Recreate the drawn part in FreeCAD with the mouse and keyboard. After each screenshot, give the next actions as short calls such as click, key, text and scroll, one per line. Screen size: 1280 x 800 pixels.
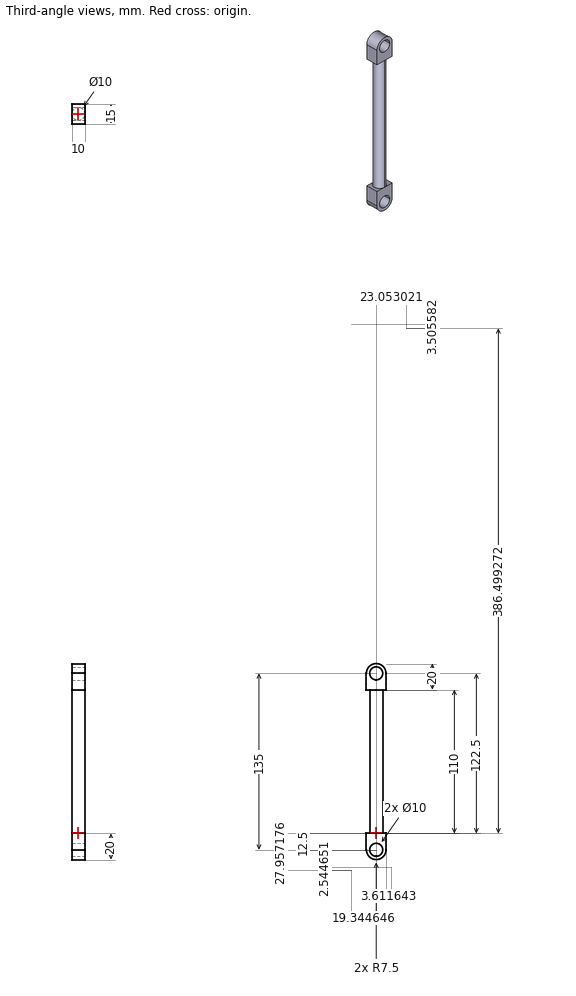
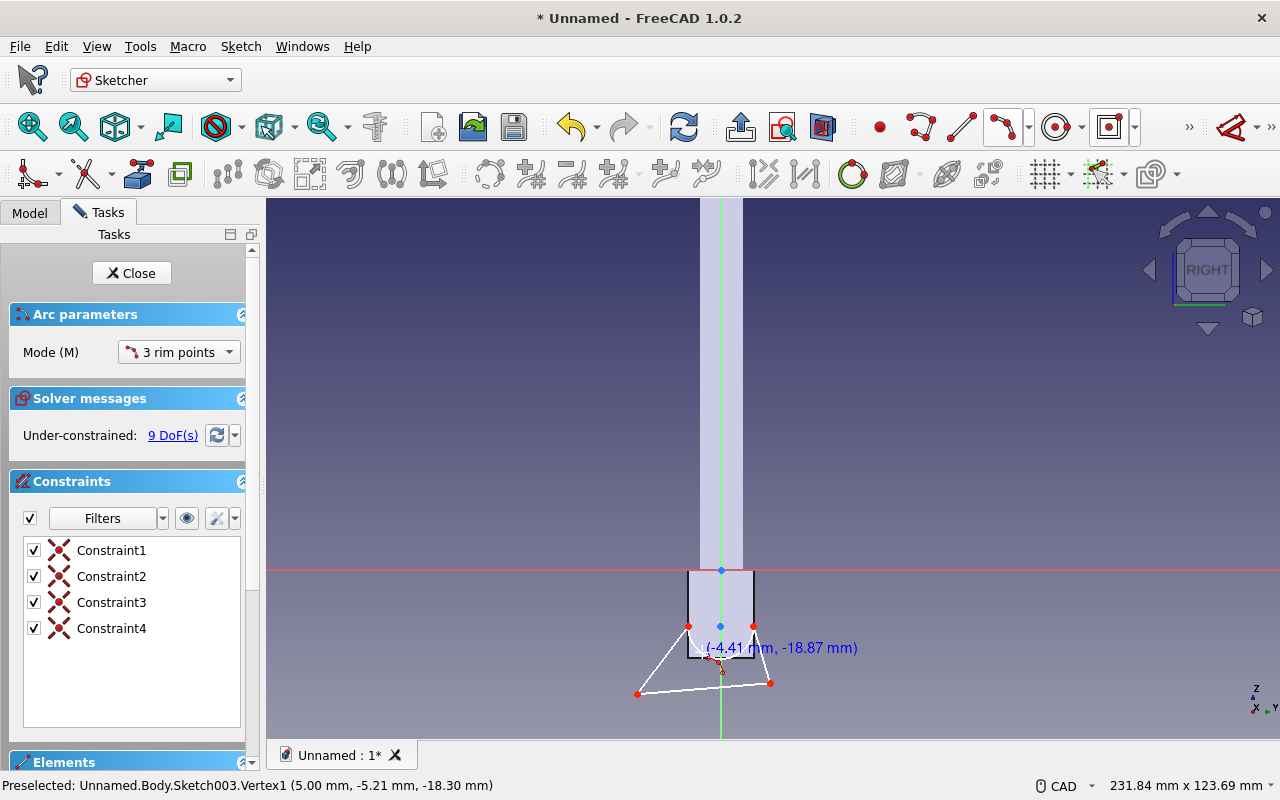
click(921, 128)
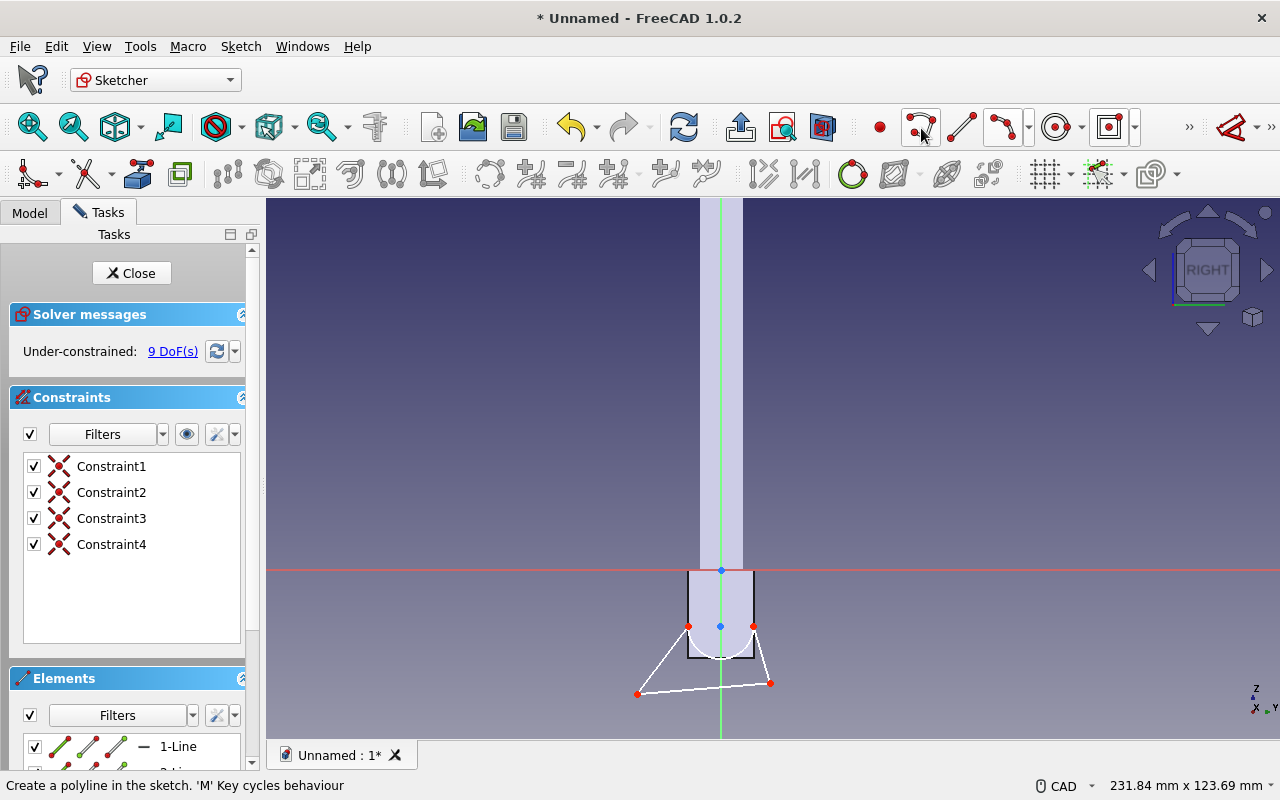
scroll(698, 643, down, 8)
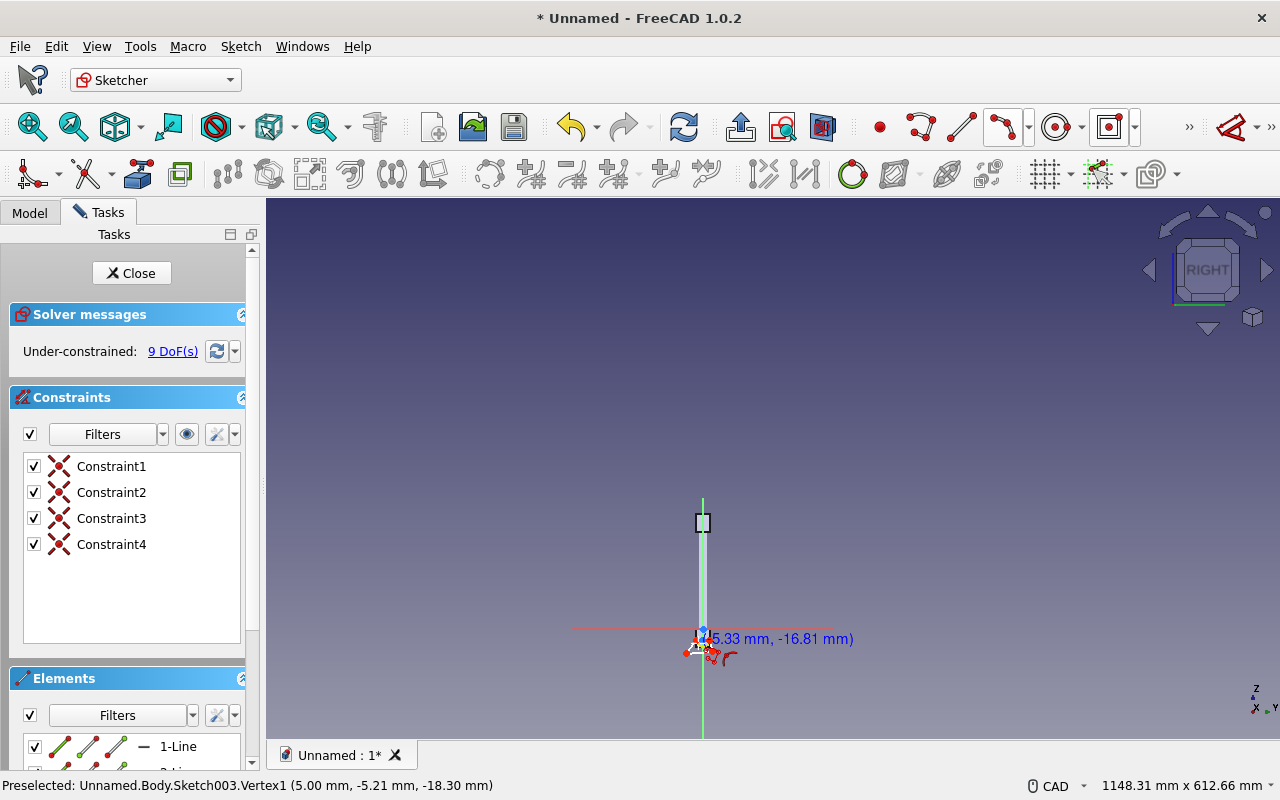
scroll(710, 521, up, 5)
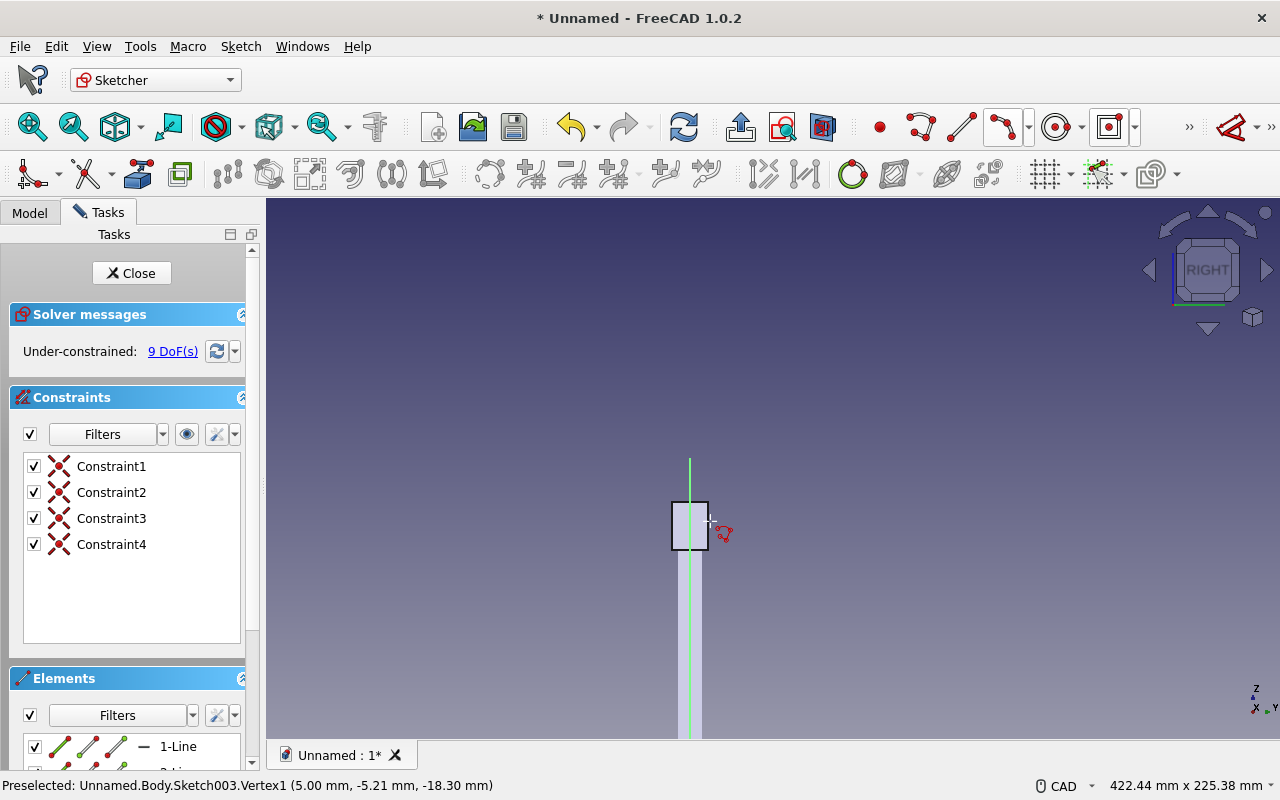
click(708, 520)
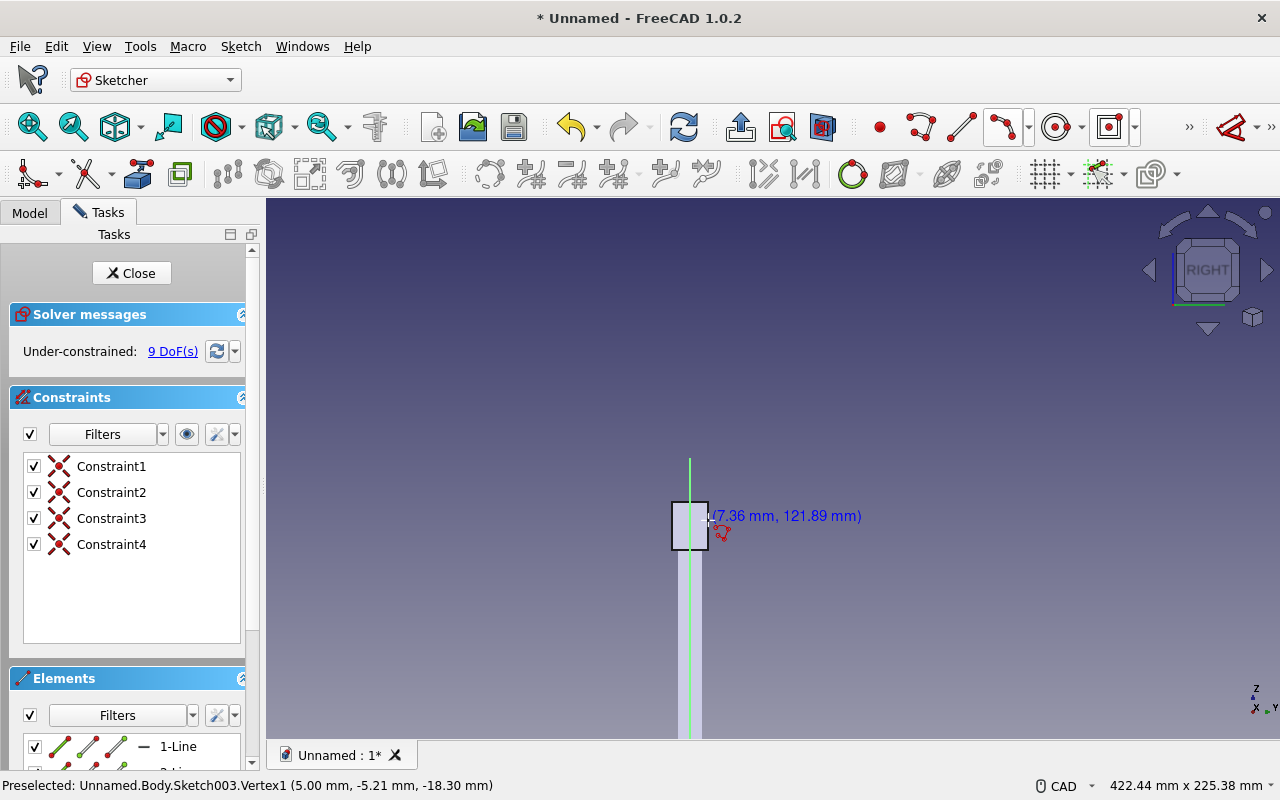
scroll(710, 521, down, 5)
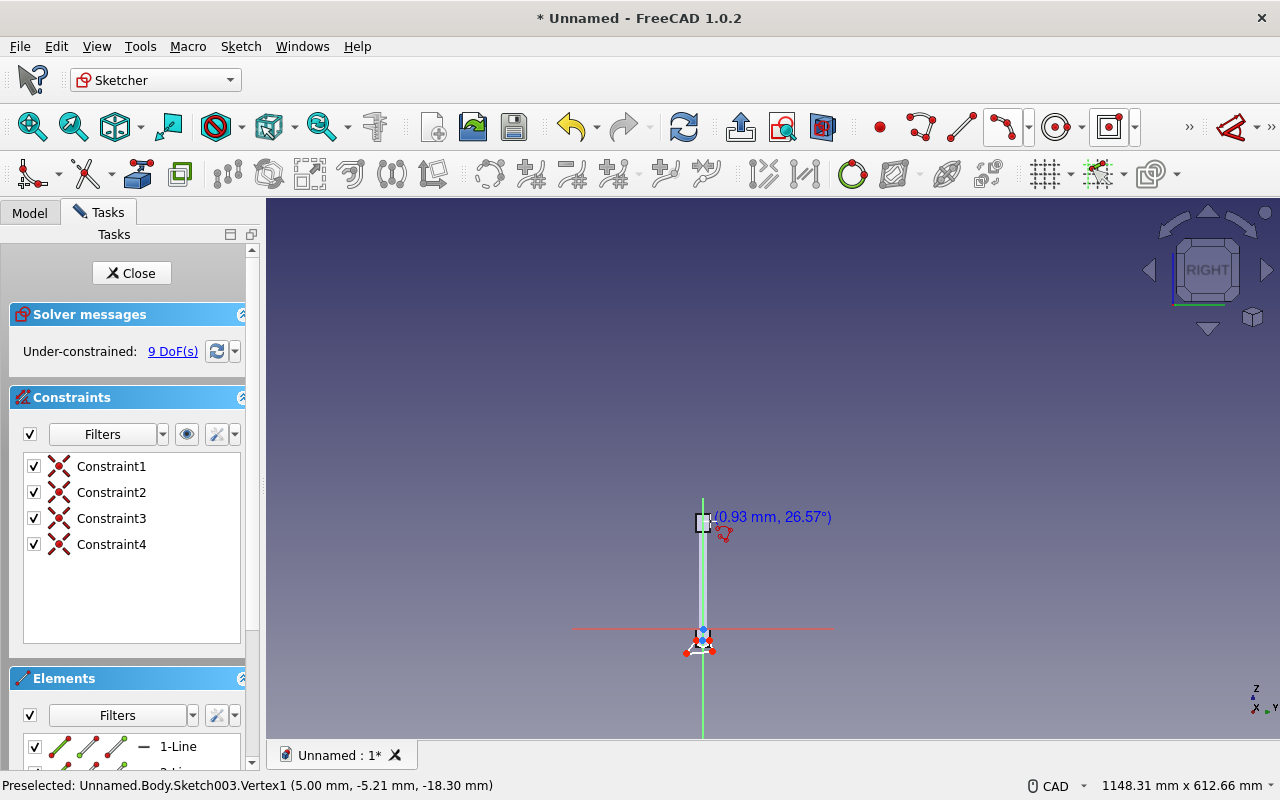
click(723, 288)
click(686, 285)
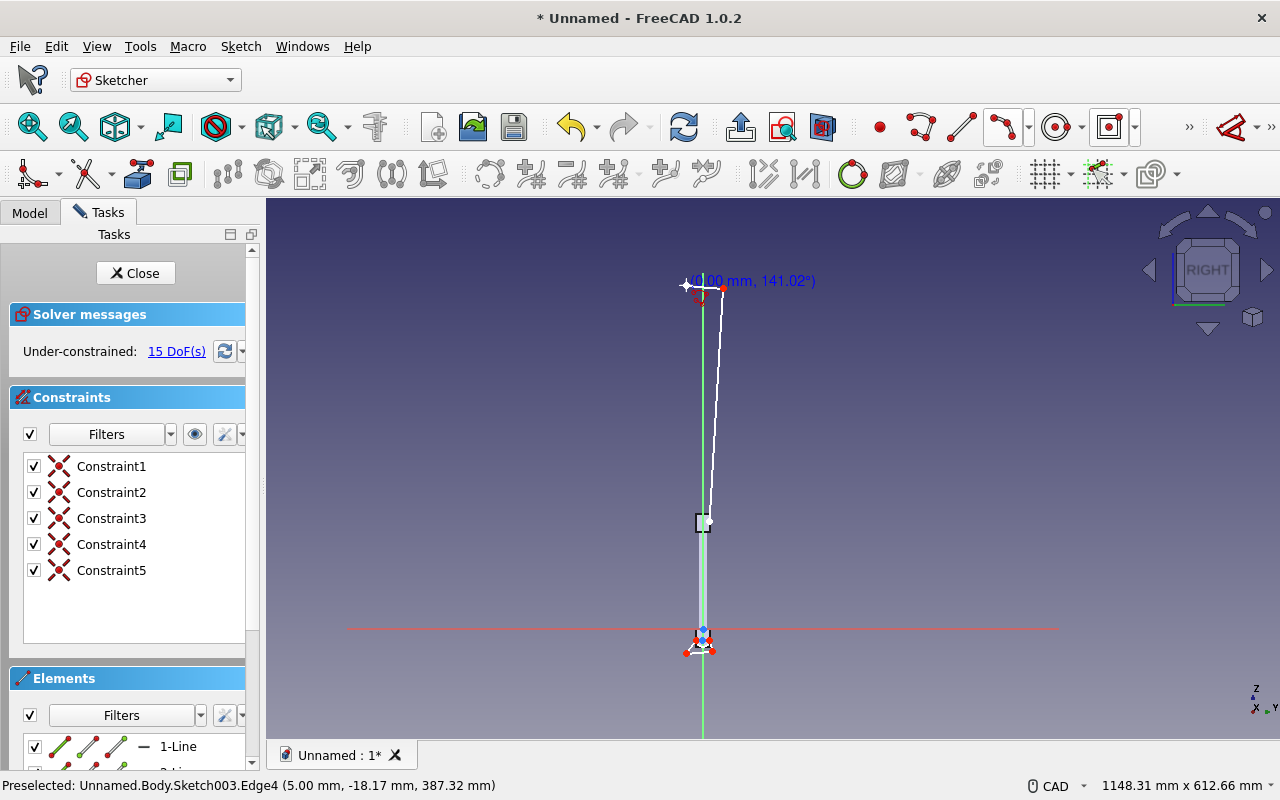
scroll(696, 521, up, 5)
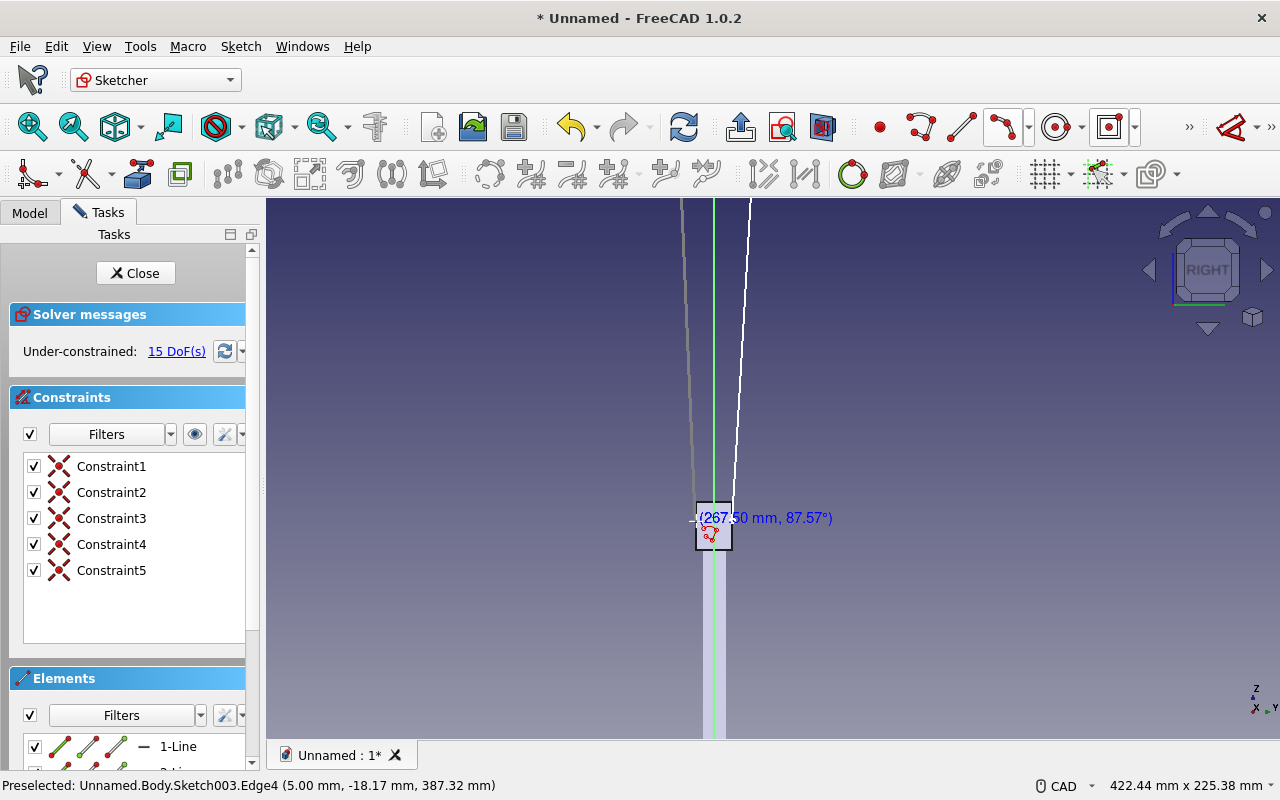
click(698, 520)
right_click(698, 520)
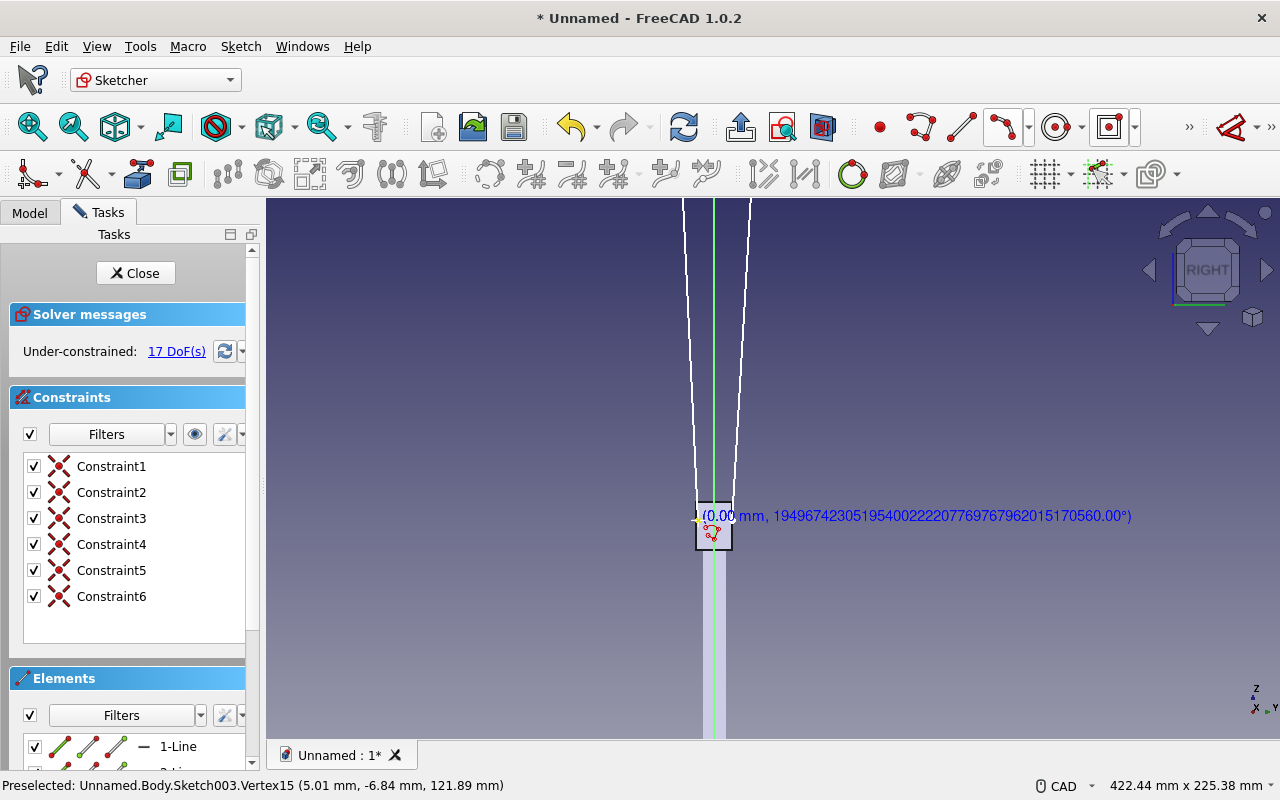
click(1002, 128)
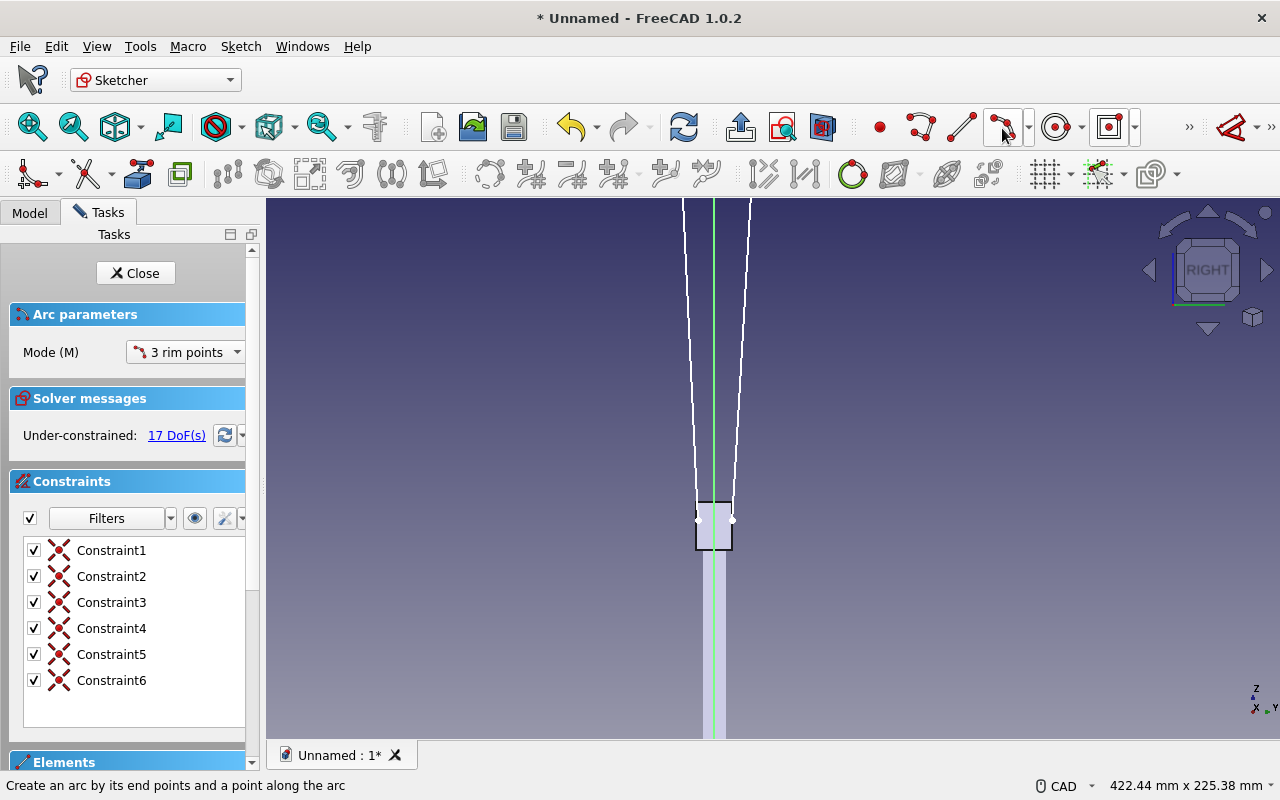
click(698, 521)
click(732, 521)